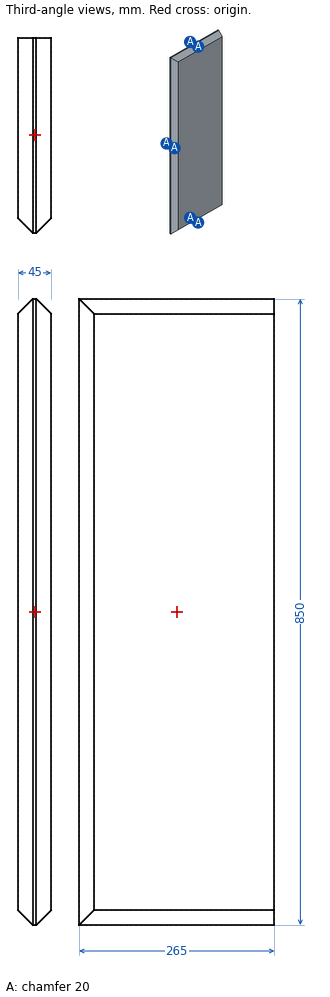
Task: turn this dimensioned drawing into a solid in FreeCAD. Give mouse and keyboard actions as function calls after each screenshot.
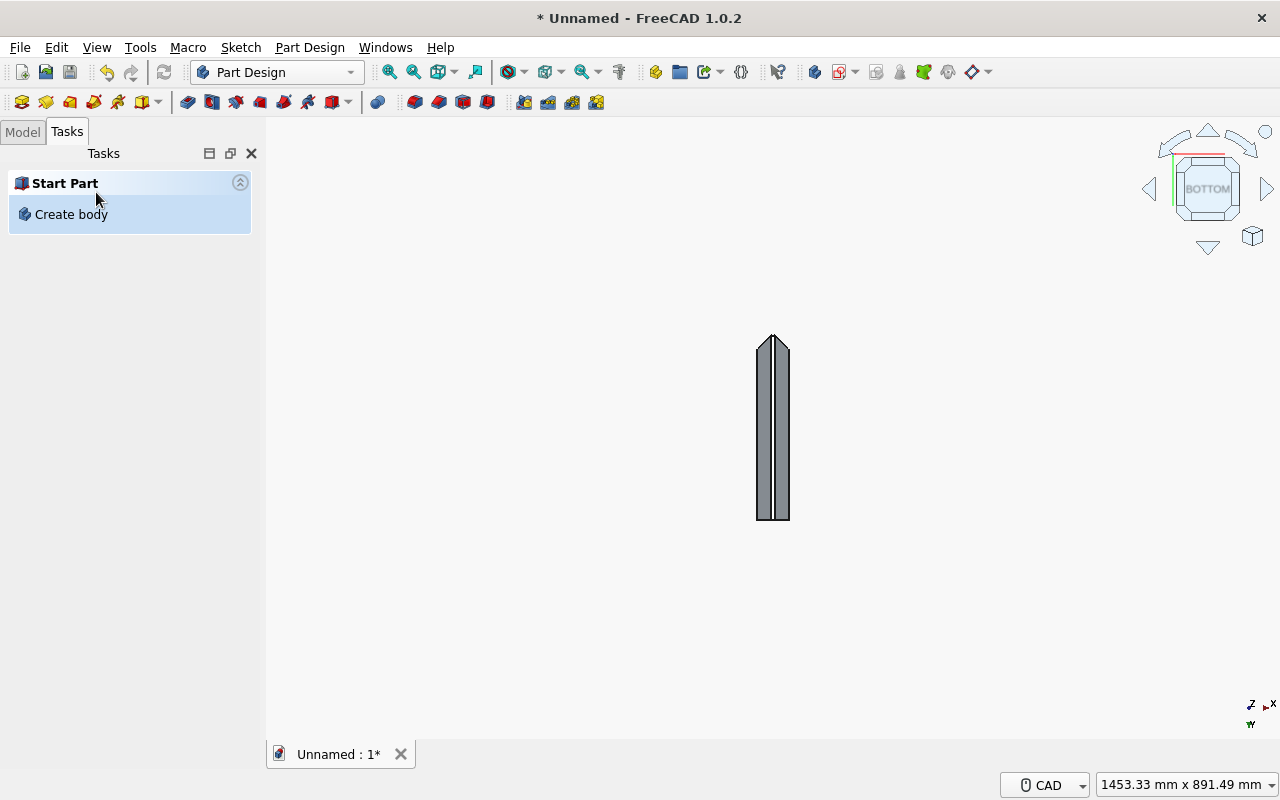
key(0)